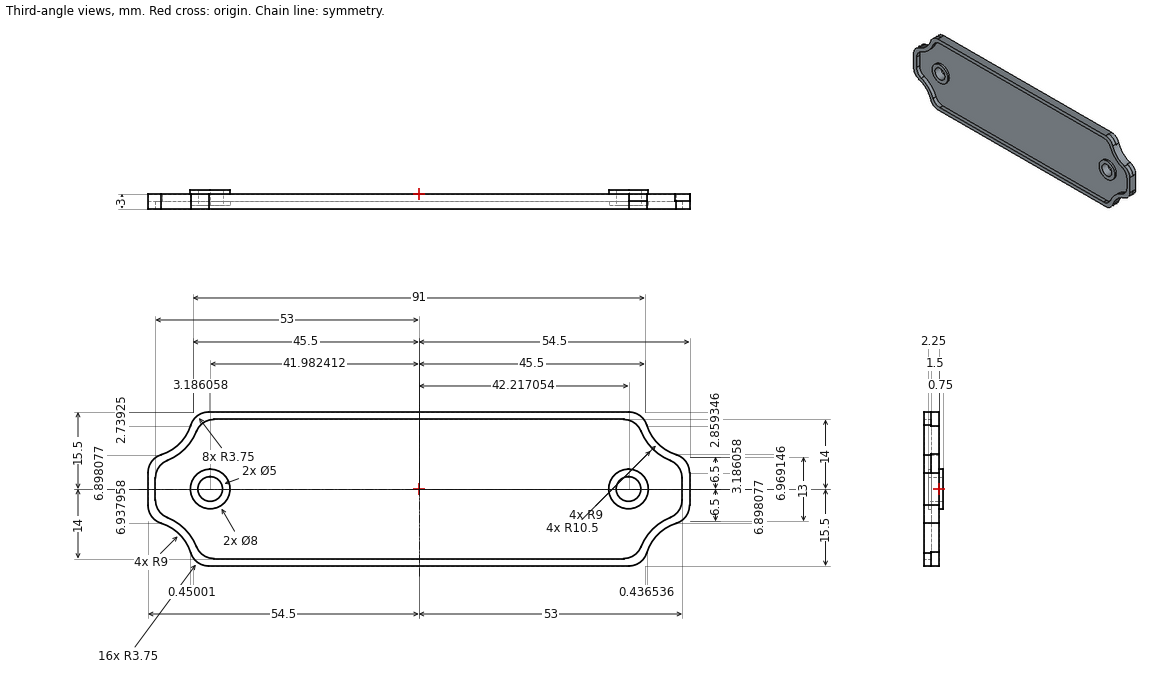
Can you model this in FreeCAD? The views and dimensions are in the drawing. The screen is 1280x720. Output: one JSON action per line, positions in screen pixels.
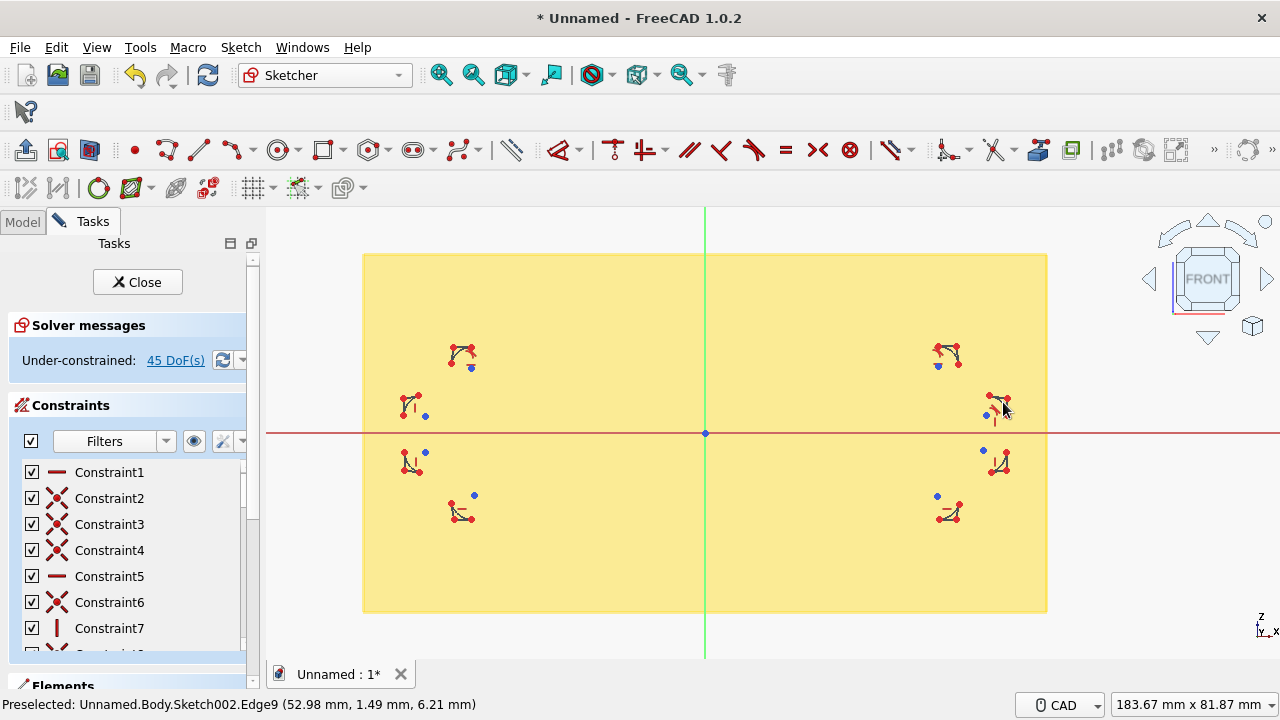
{"action": "scroll", "coordinate": [1007, 465], "scroll_direction": "up", "scroll_amount": 7}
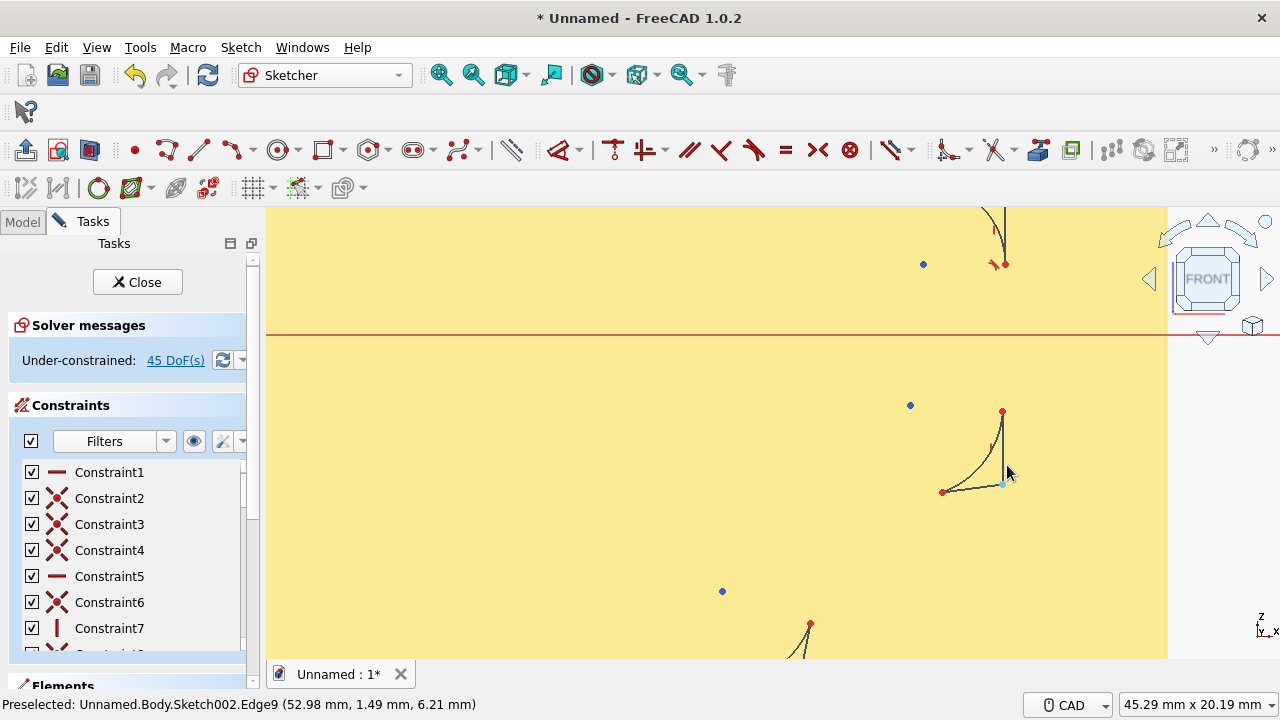
{"action": "left_click", "coordinate": [1003, 462]}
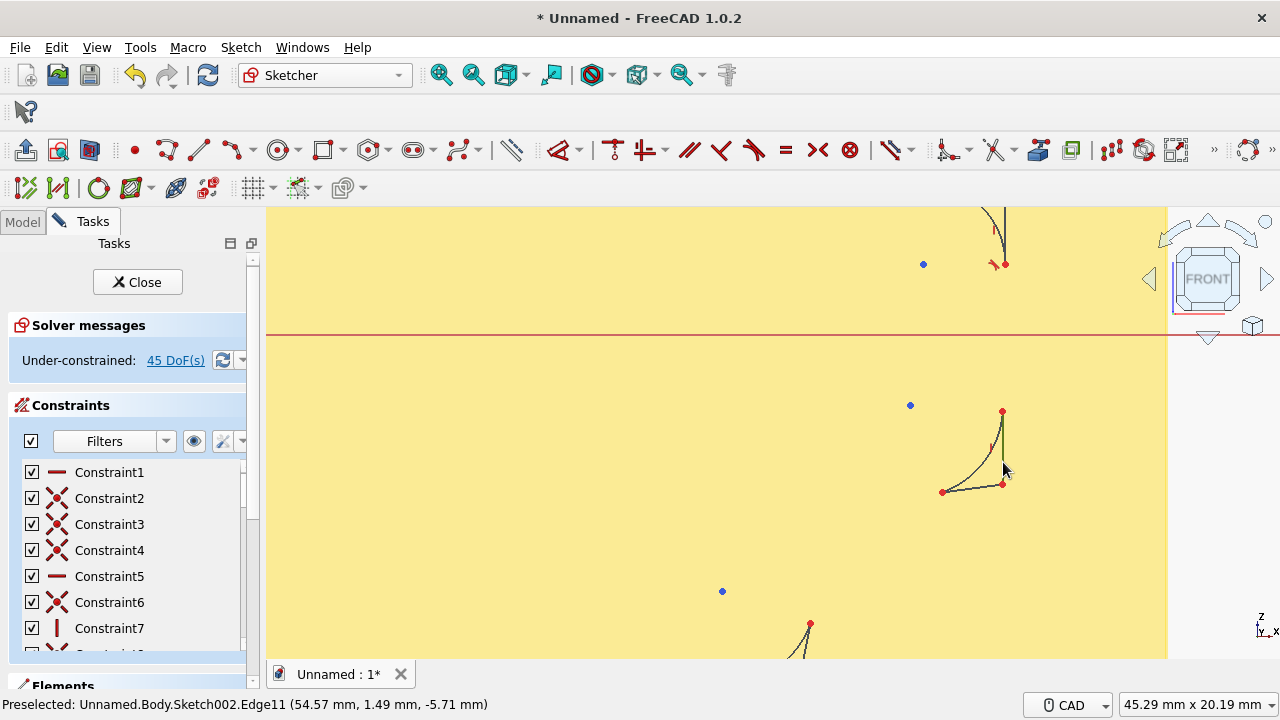
{"action": "left_click", "coordinate": [970, 477]}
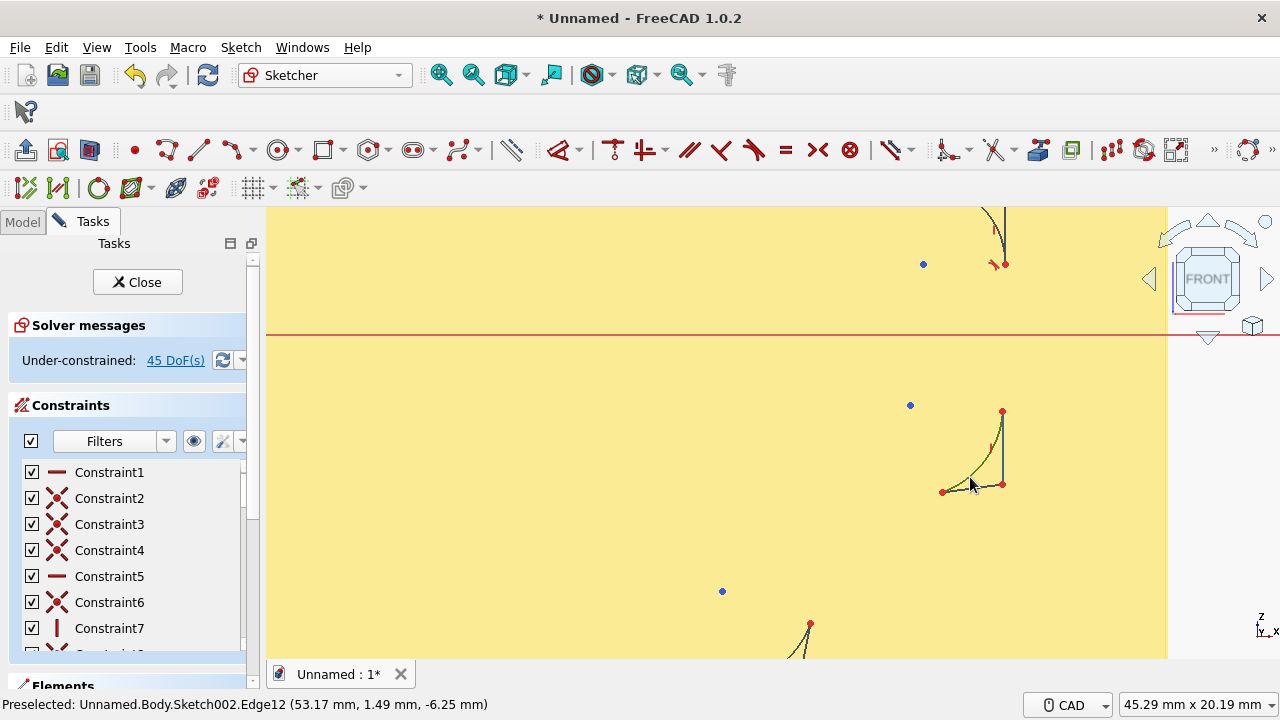
{"action": "left_click", "coordinate": [754, 150]}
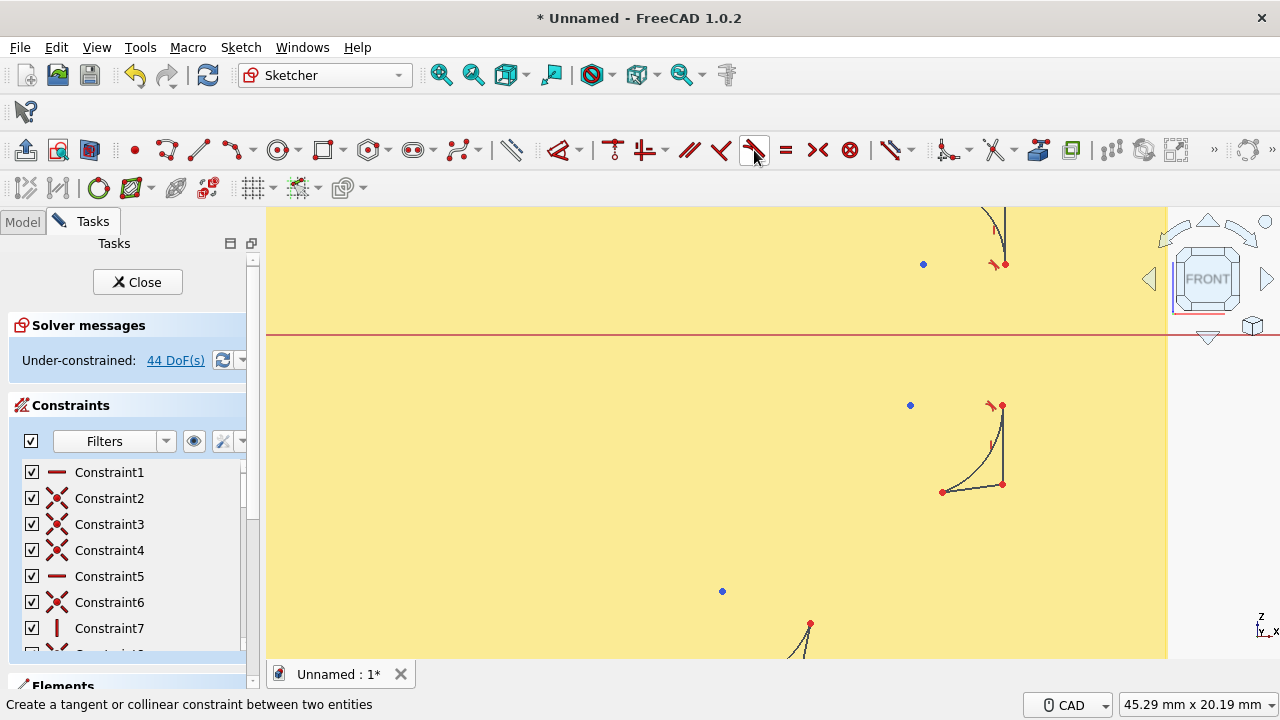
{"action": "scroll", "coordinate": [1007, 465], "scroll_direction": "down", "scroll_amount": 7}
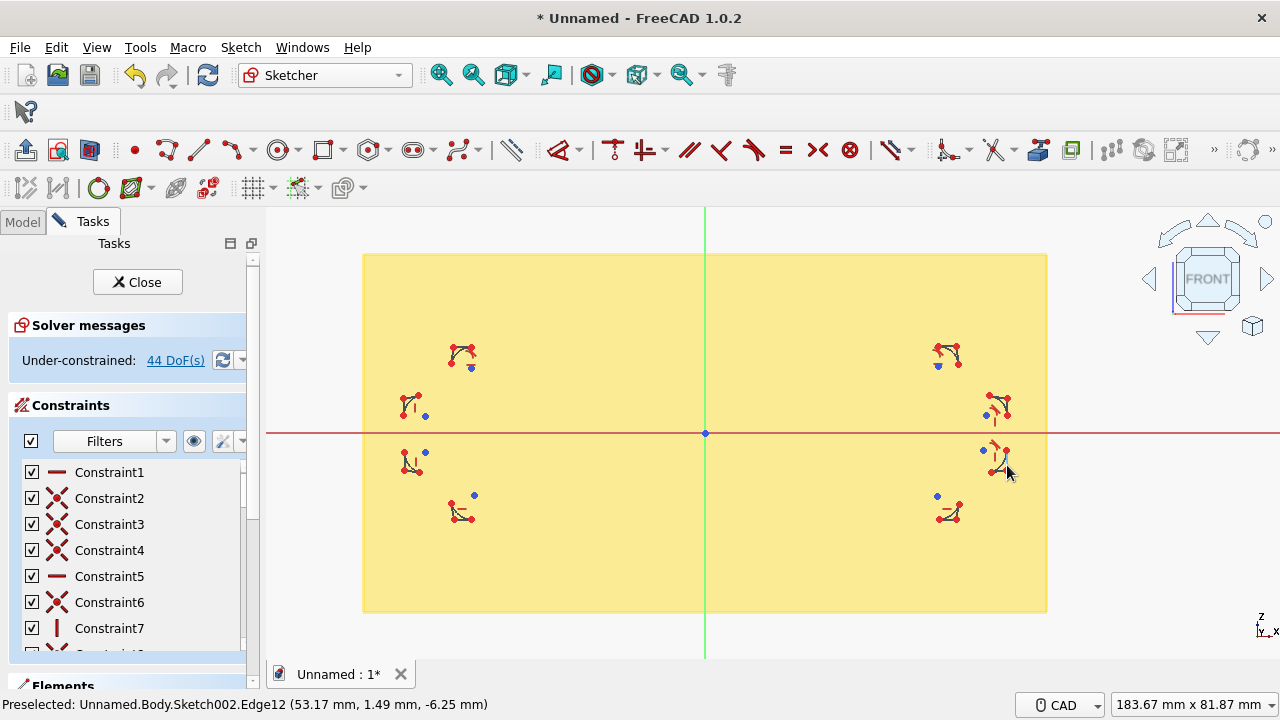
{"action": "scroll", "coordinate": [951, 520], "scroll_direction": "up", "scroll_amount": 7}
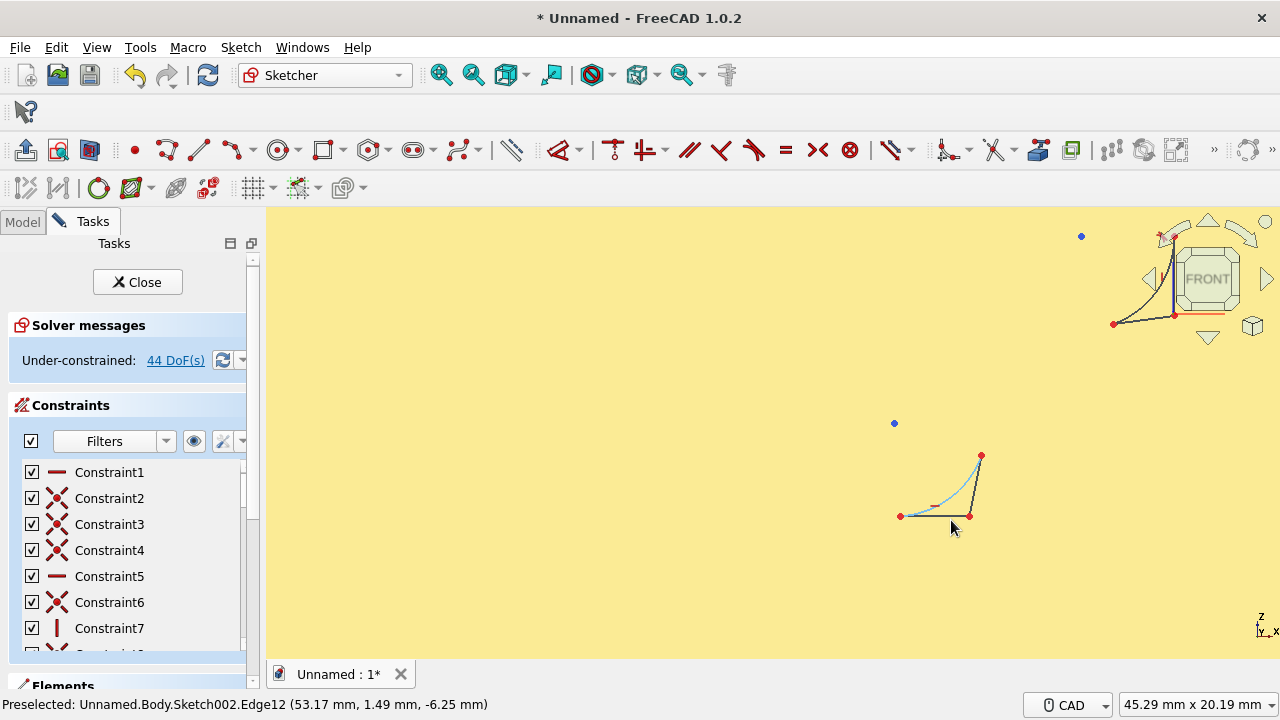
{"action": "left_click", "coordinate": [949, 516]}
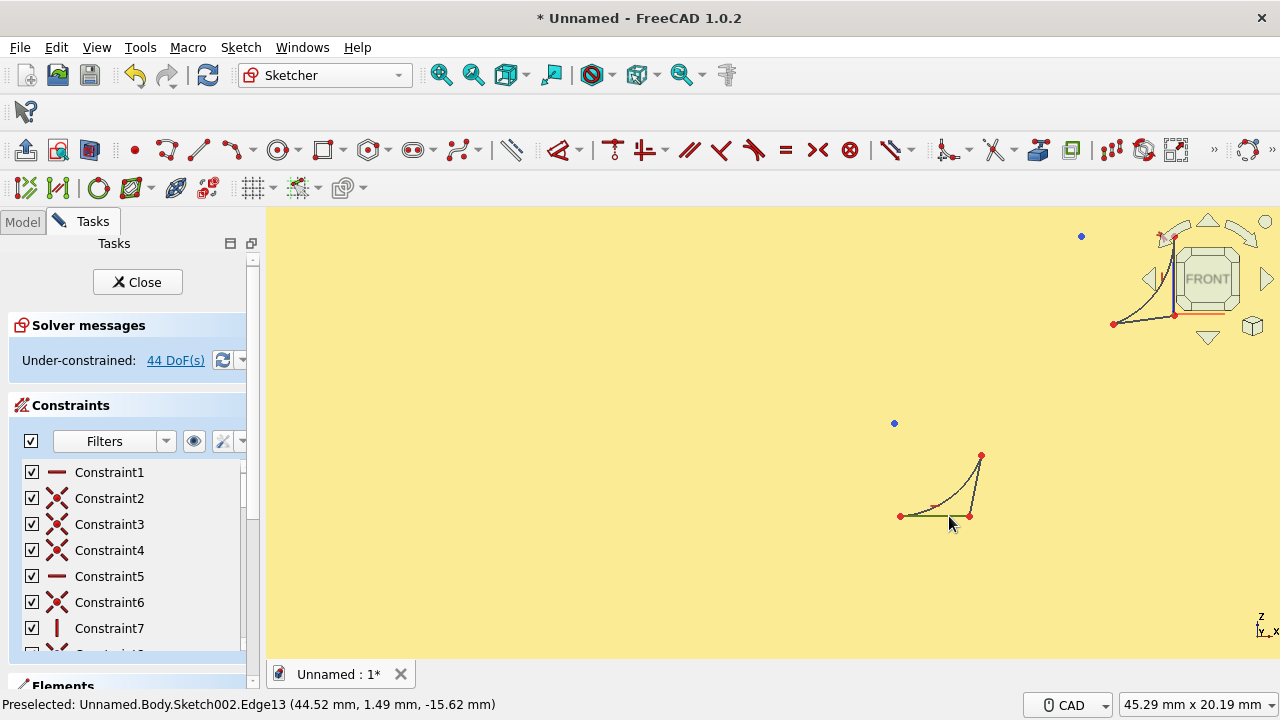
{"action": "scroll", "coordinate": [966, 483], "scroll_direction": "up", "scroll_amount": 2}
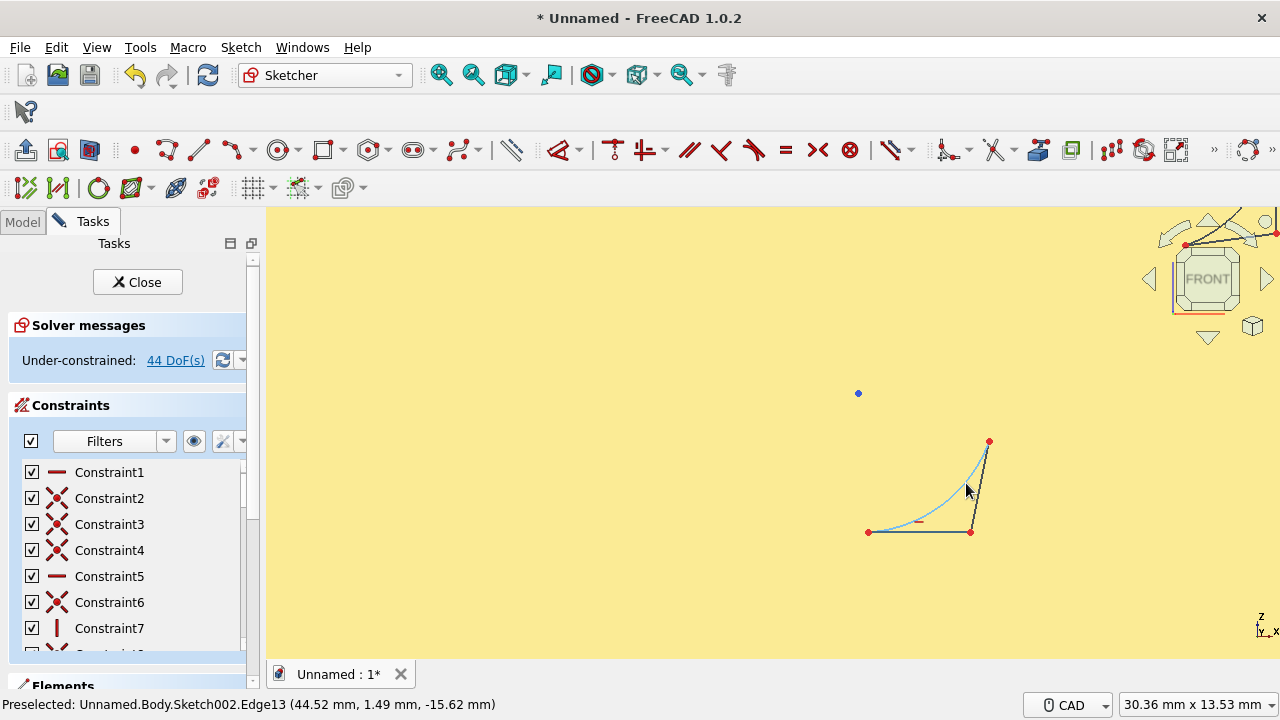
{"action": "left_click", "coordinate": [965, 483]}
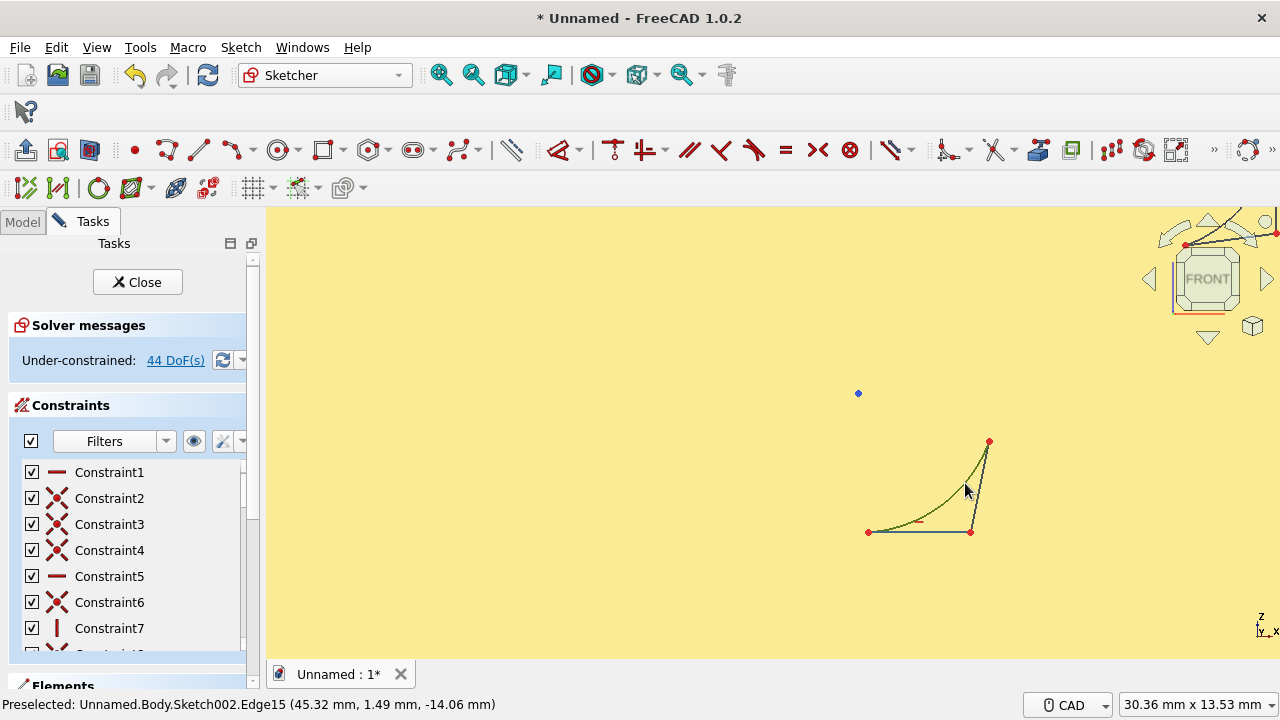
{"action": "left_click", "coordinate": [754, 150]}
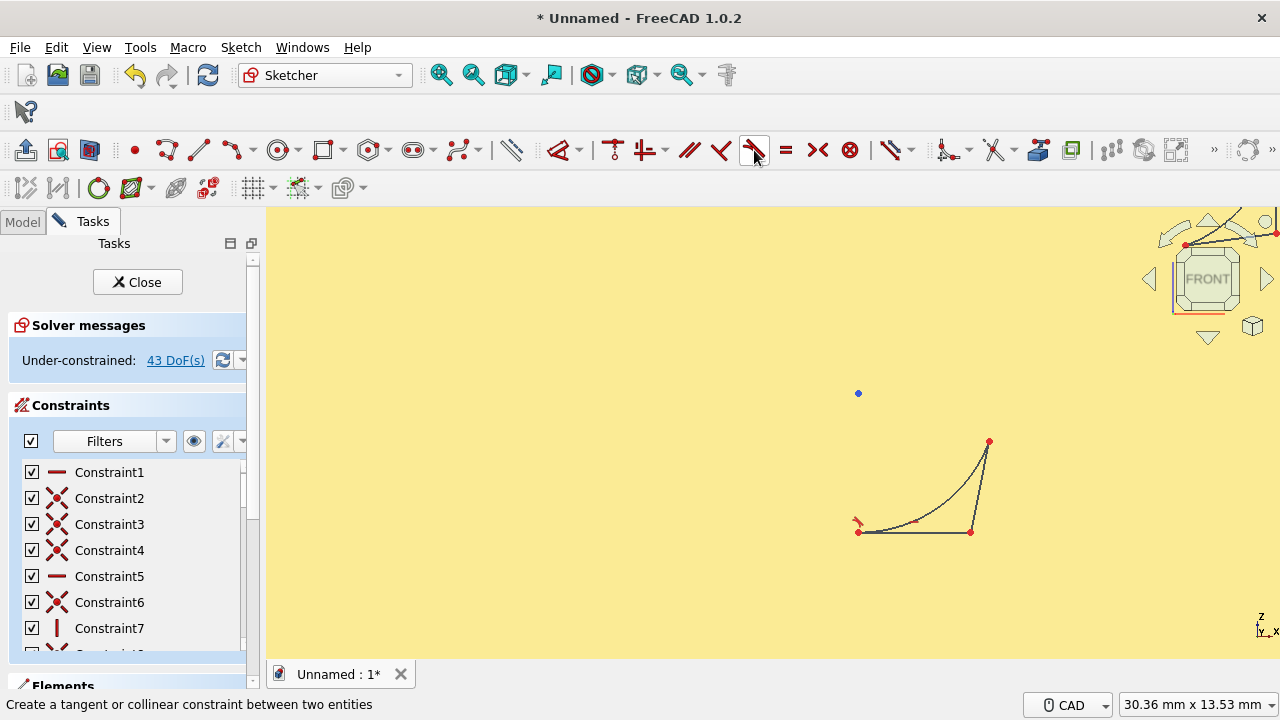
{"action": "scroll", "coordinate": [952, 517], "scroll_direction": "down", "scroll_amount": 9}